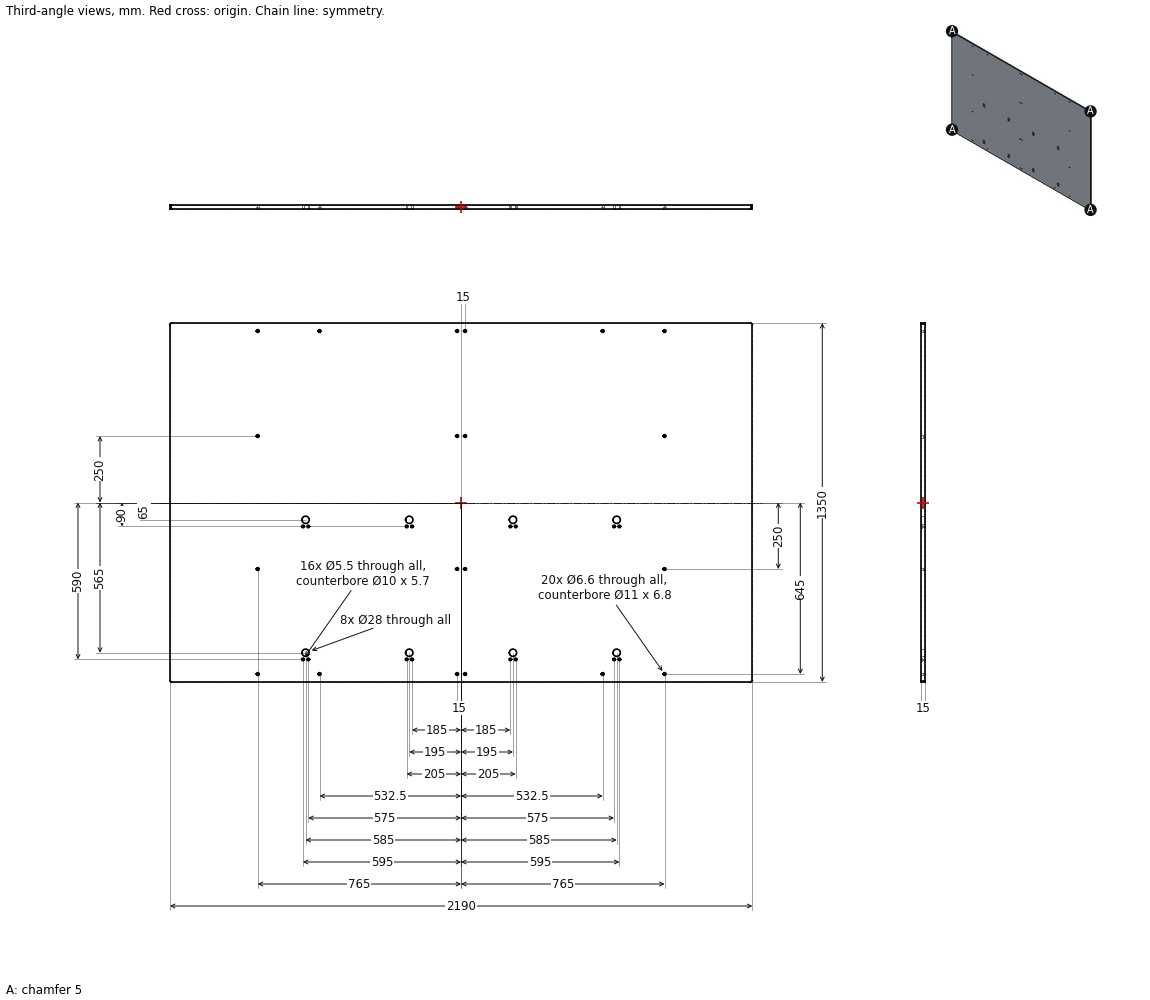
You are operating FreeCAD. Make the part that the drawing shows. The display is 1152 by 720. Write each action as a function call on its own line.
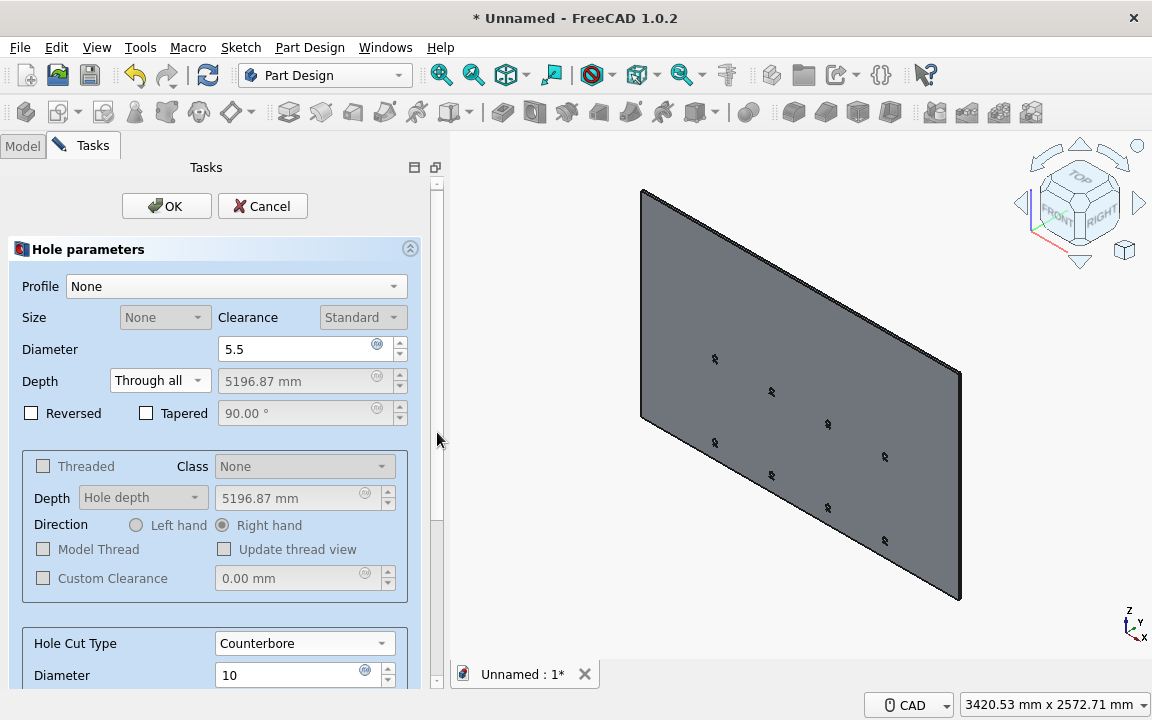
click(167, 206)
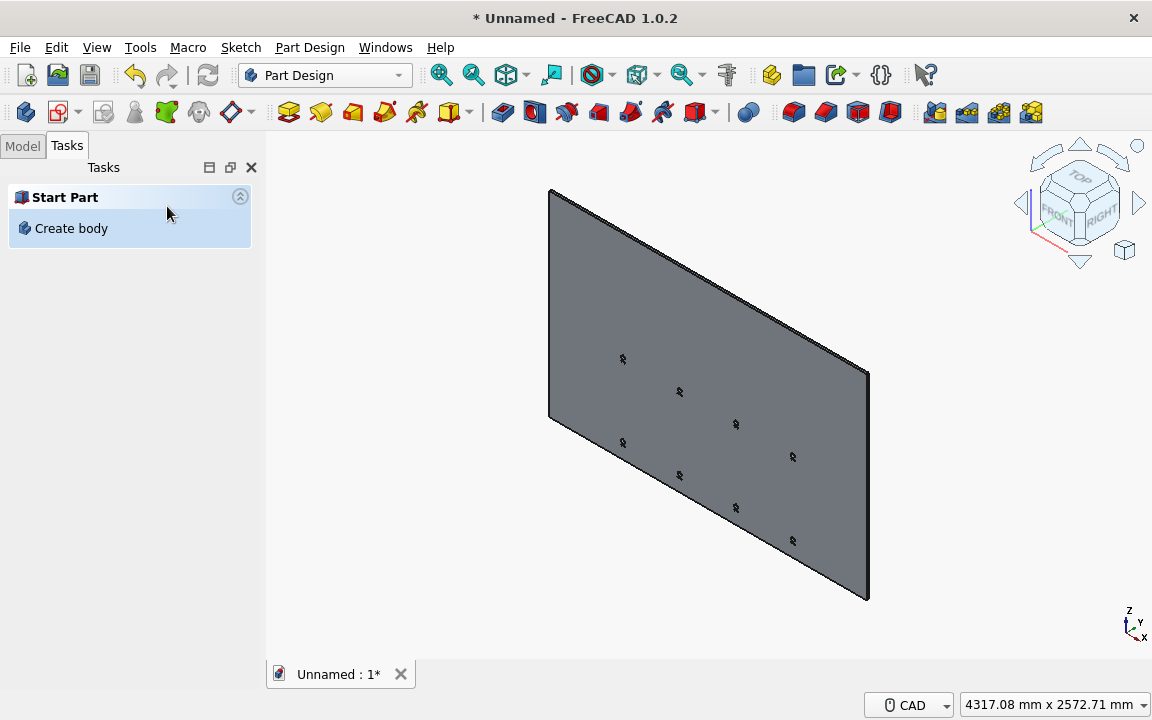
click(708, 362)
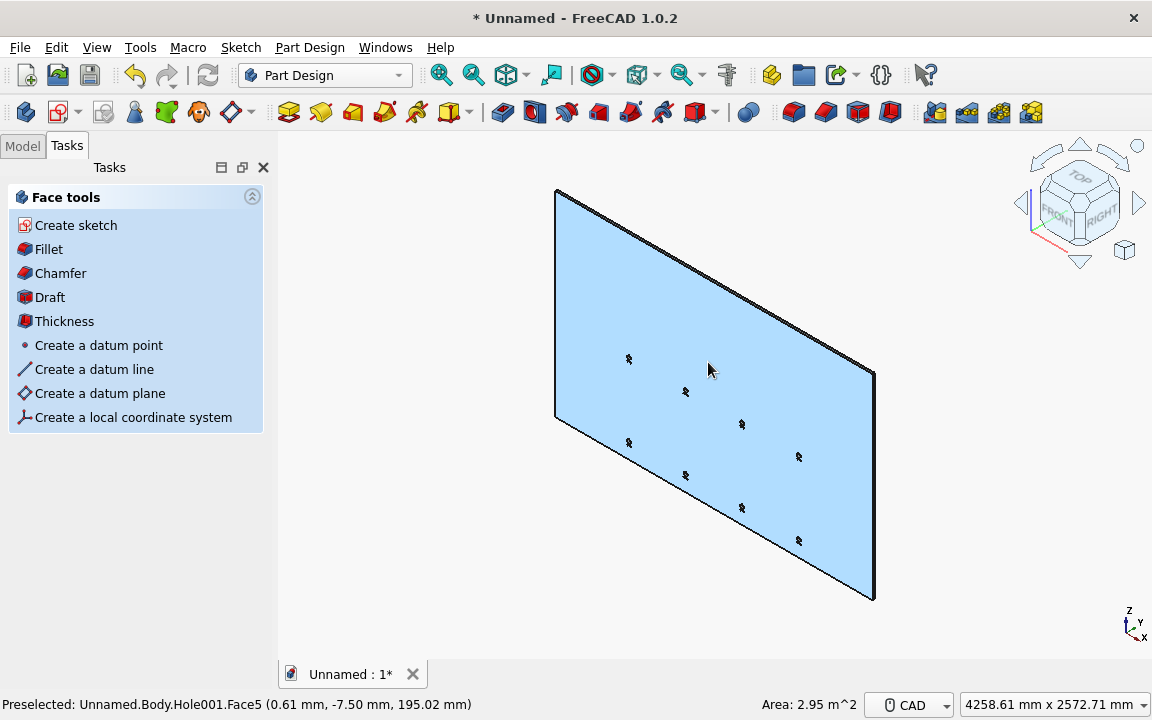
click(58, 112)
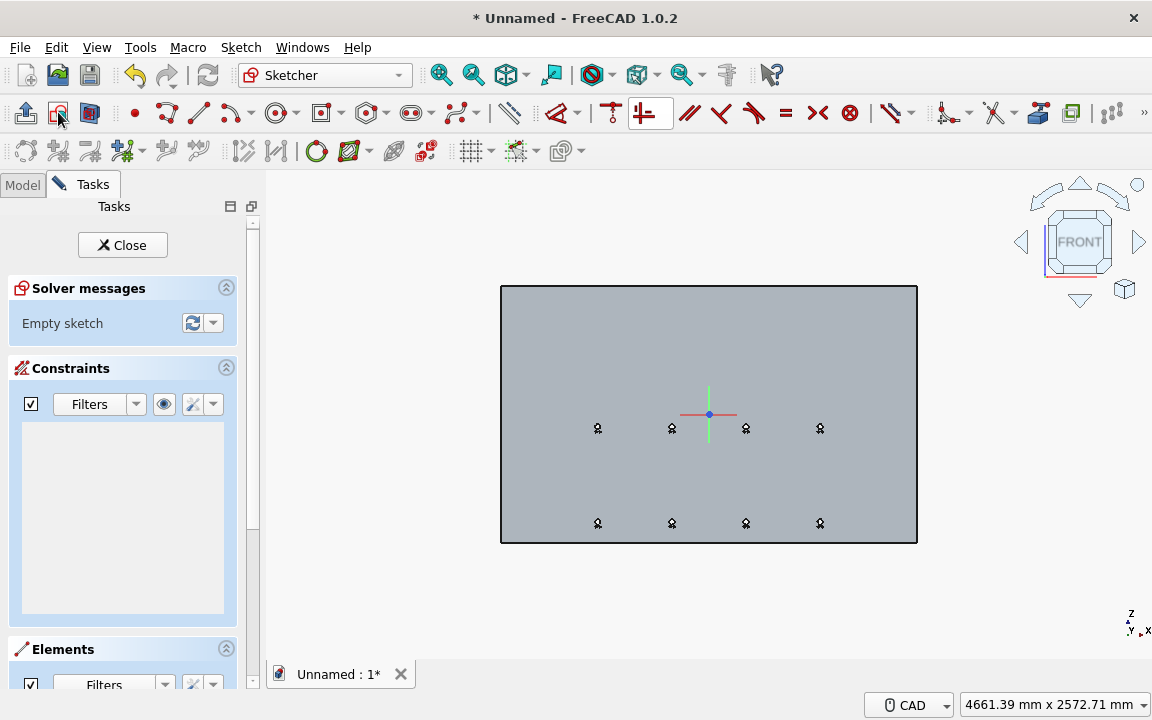
key(g)
key(c)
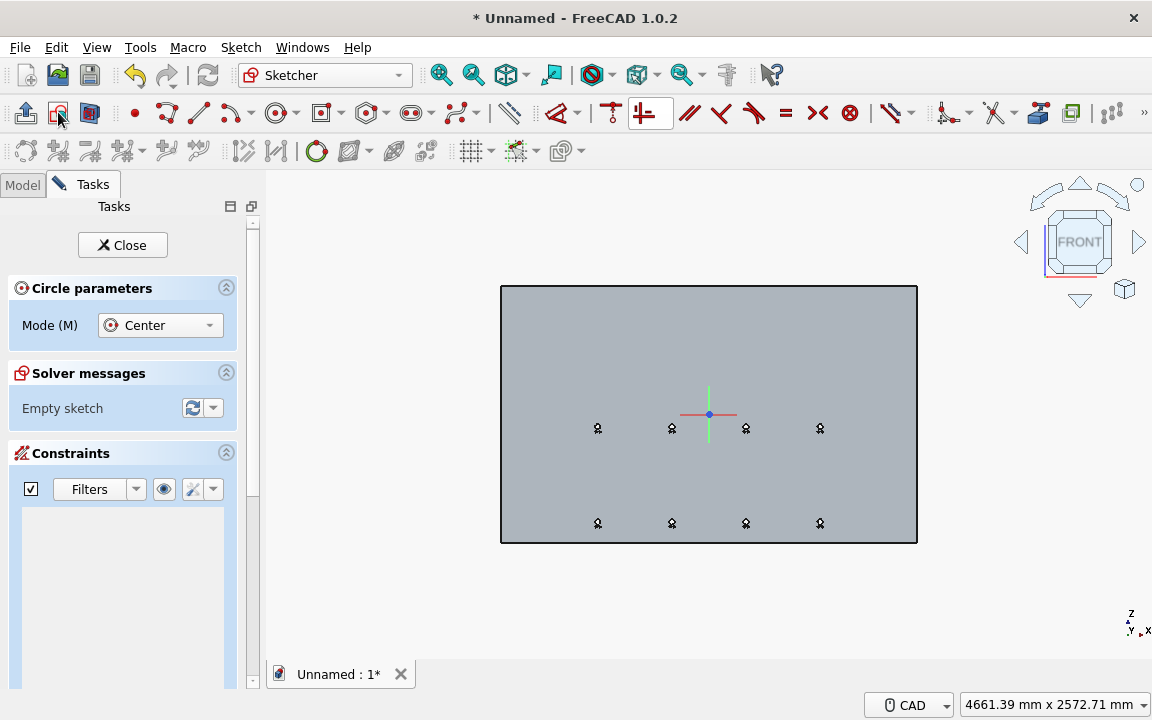
scroll(854, 537, up, 18)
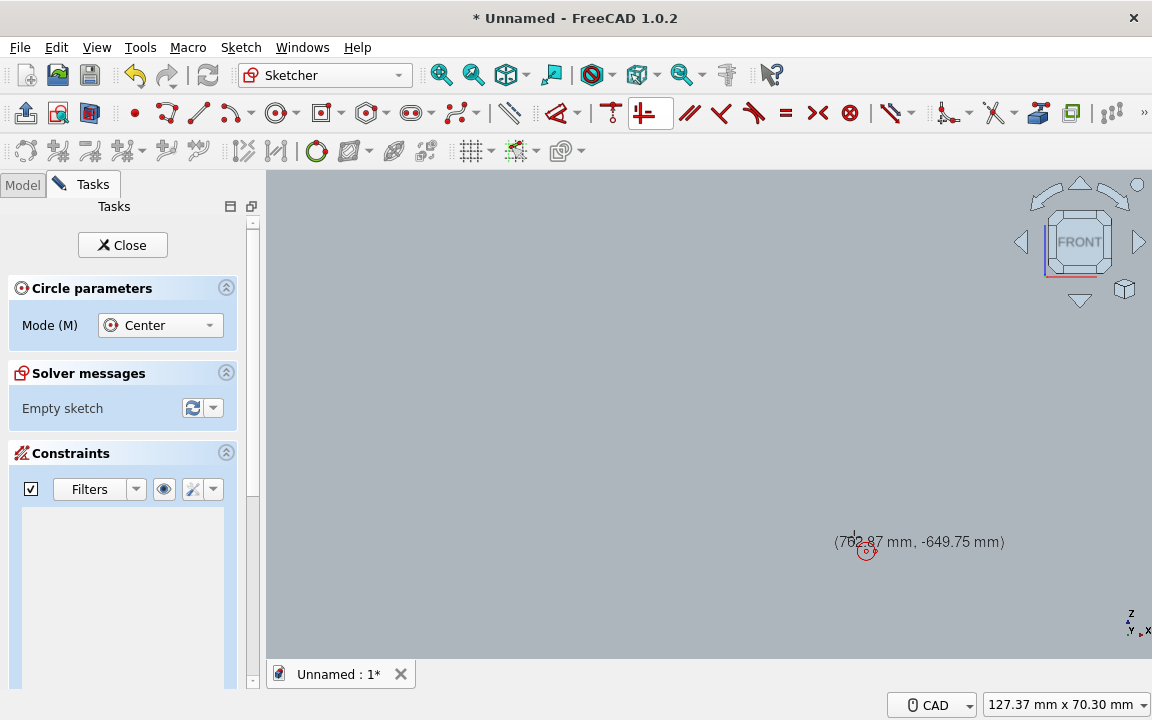
scroll(858, 601, down, 16)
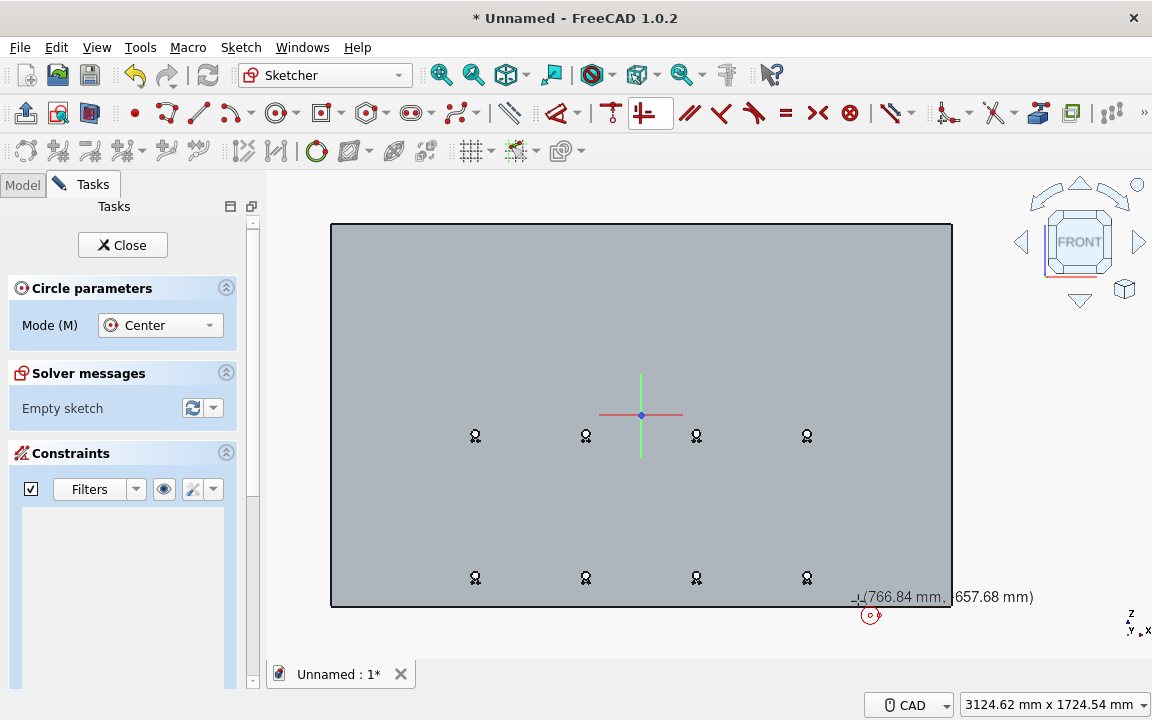
click(858, 598)
move(859, 598)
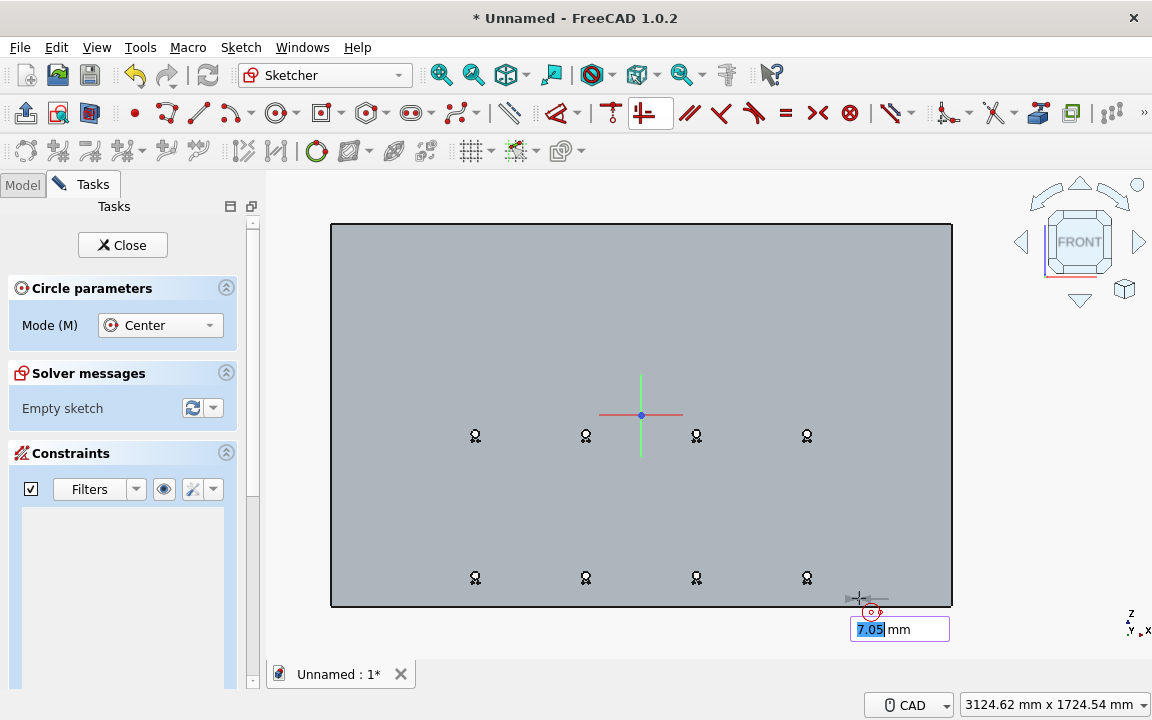
text(6.6)
key(Return)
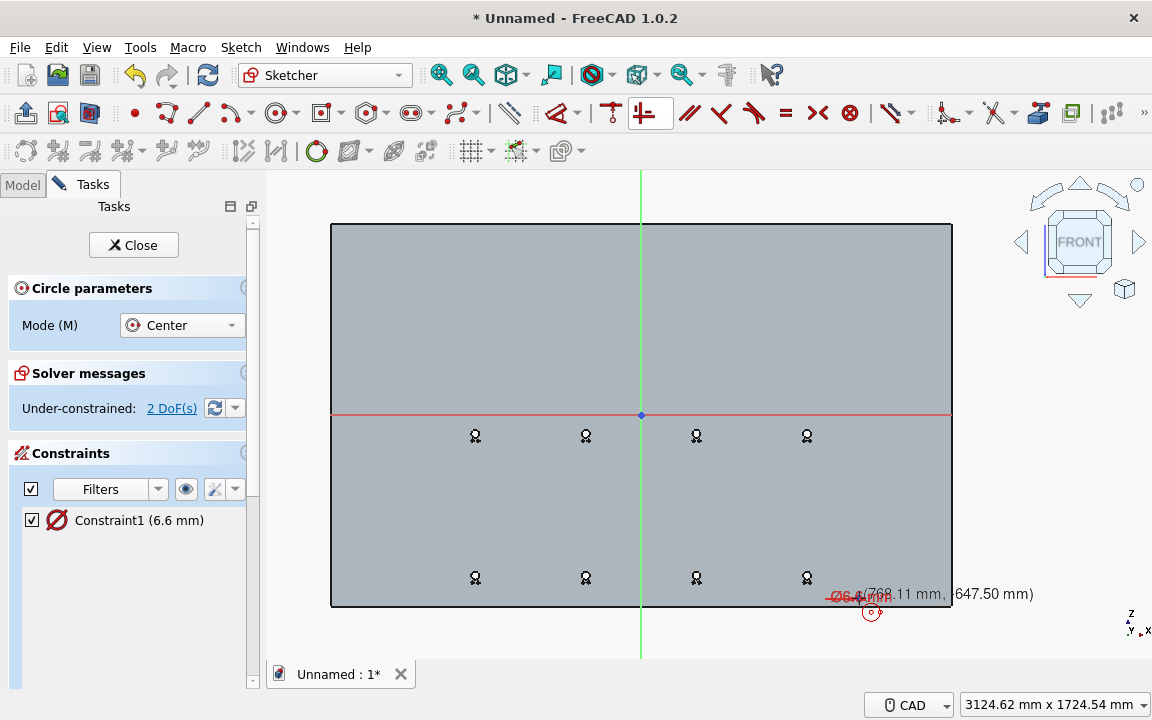
scroll(792, 598, up, 16)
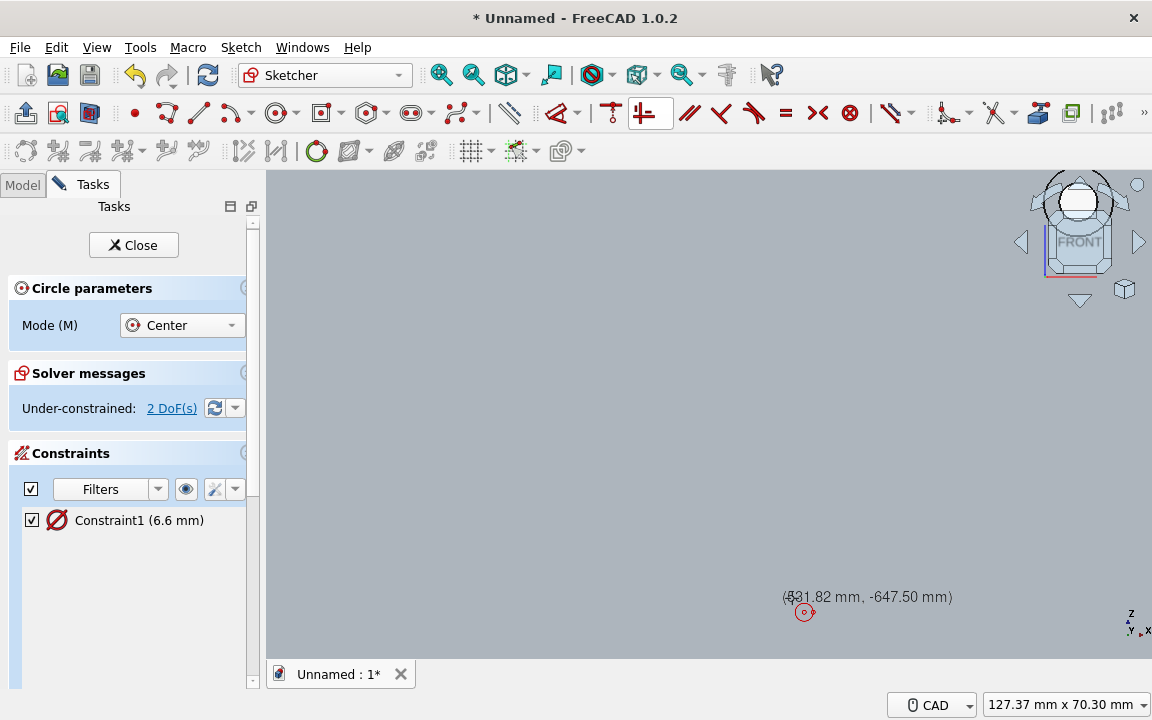
scroll(792, 598, down, 16)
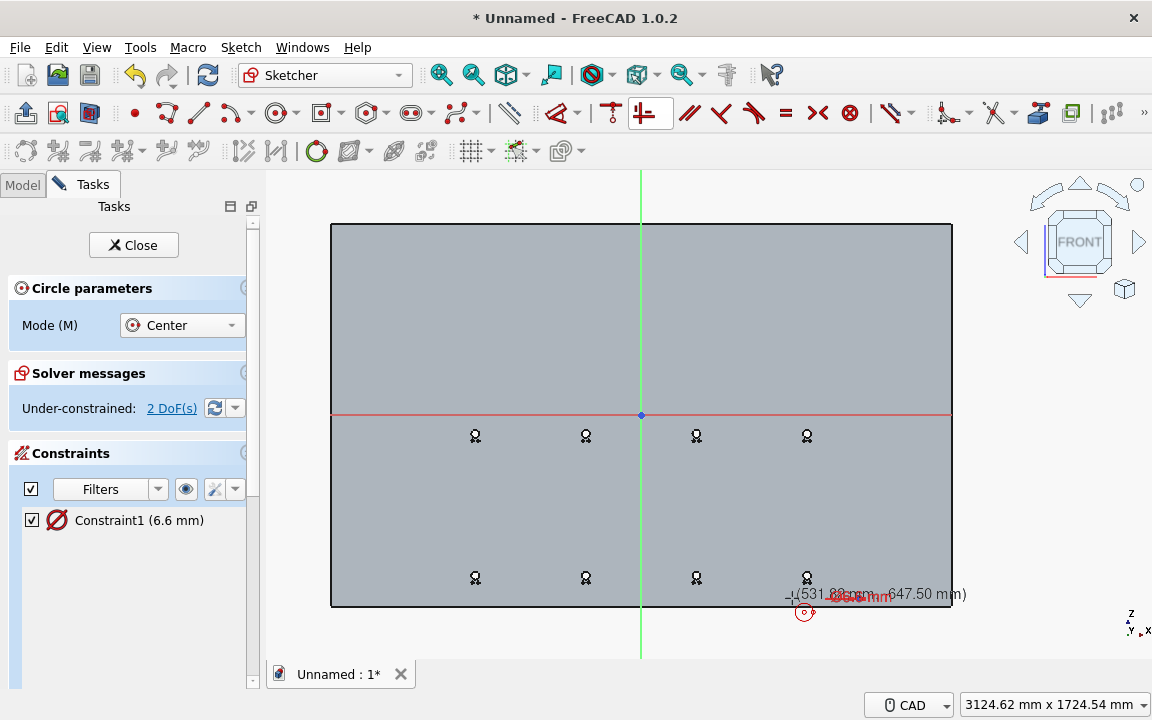
click(792, 598)
move(793, 598)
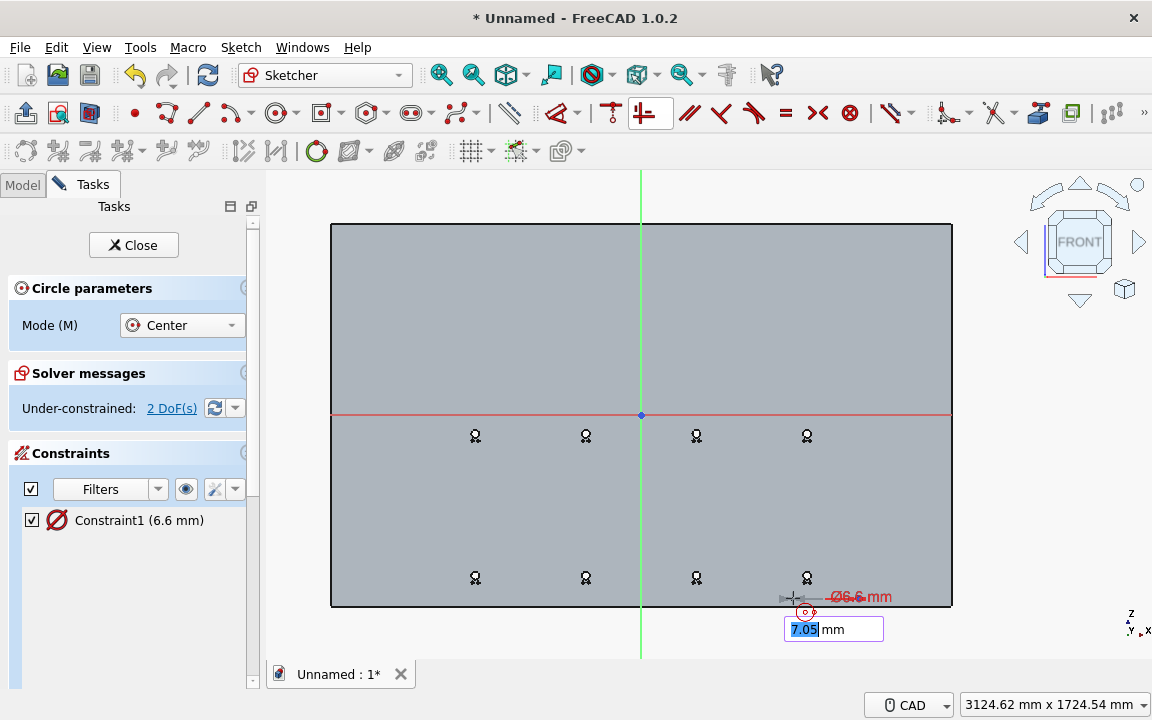
text(6.6)
key(Return)